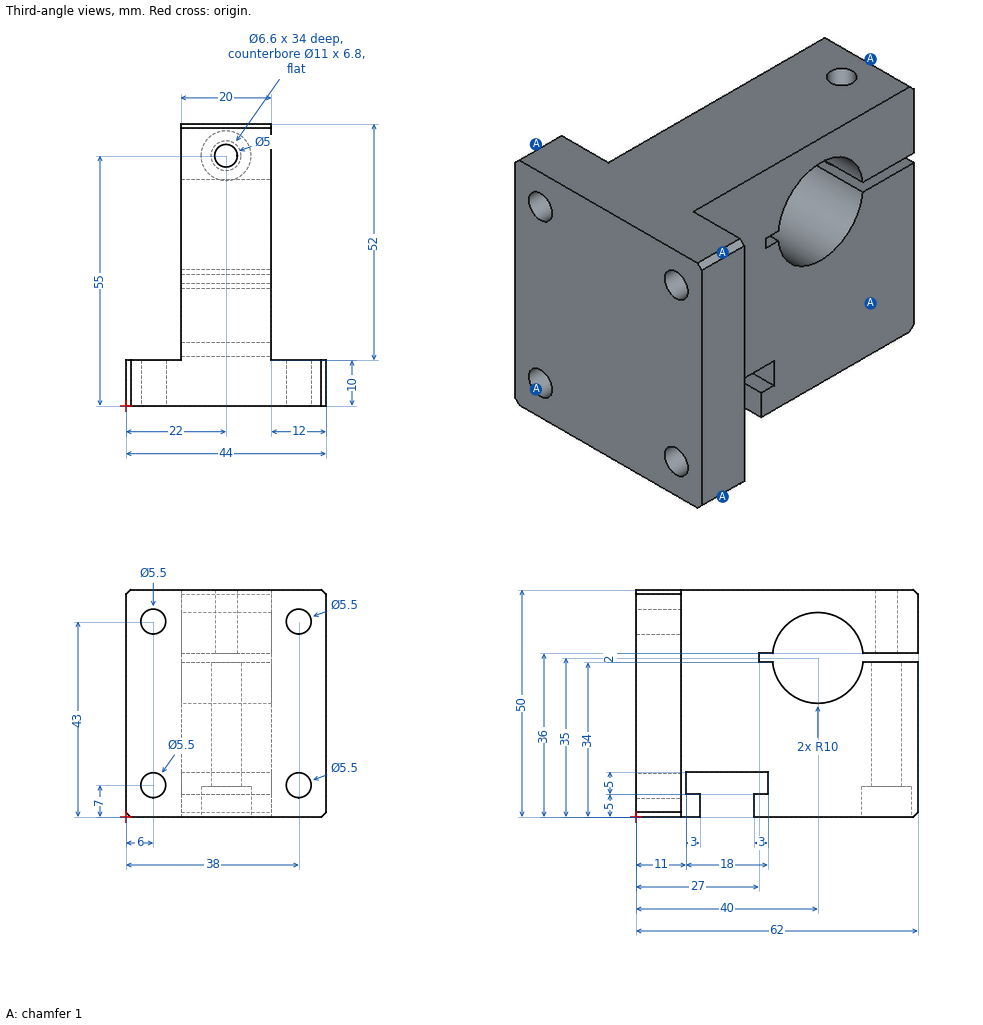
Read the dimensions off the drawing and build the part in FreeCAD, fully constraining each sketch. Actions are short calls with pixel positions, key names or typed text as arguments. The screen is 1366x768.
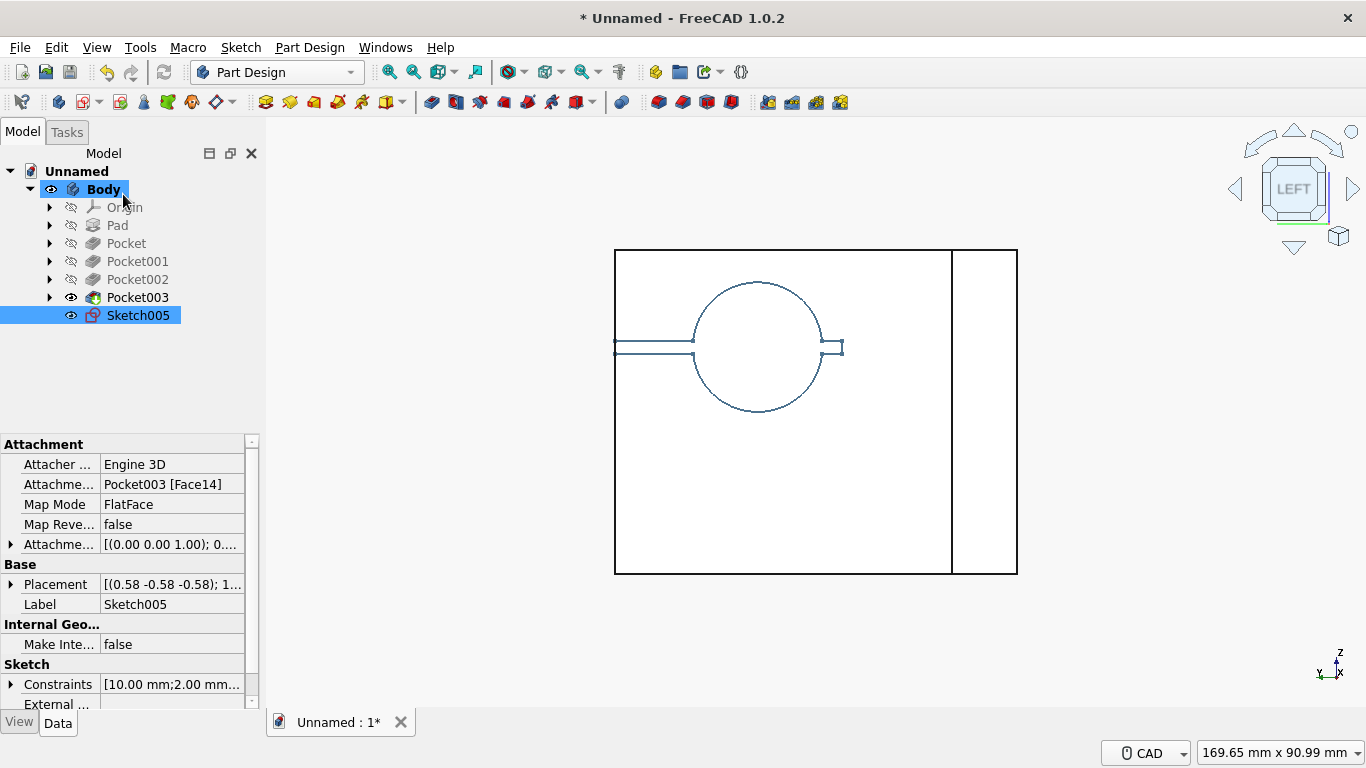
click(432, 102)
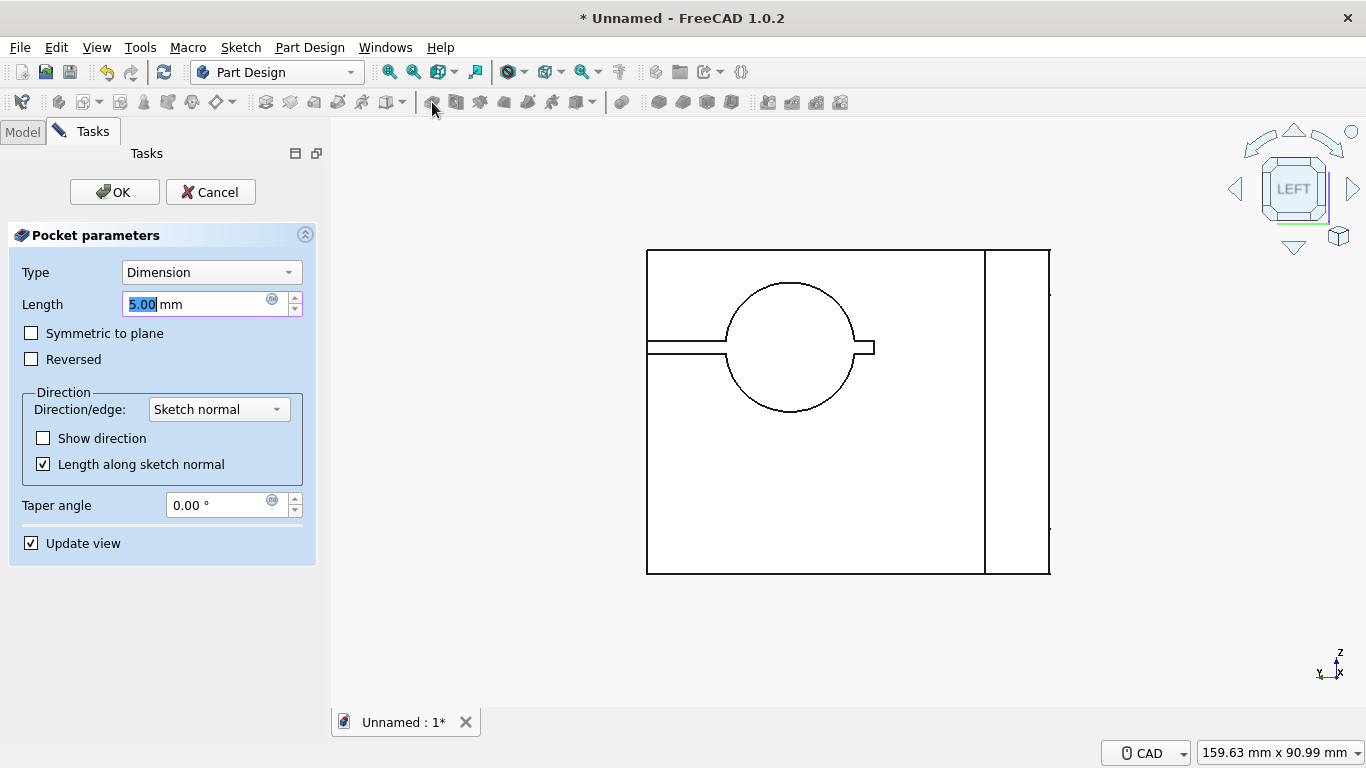
click(212, 272)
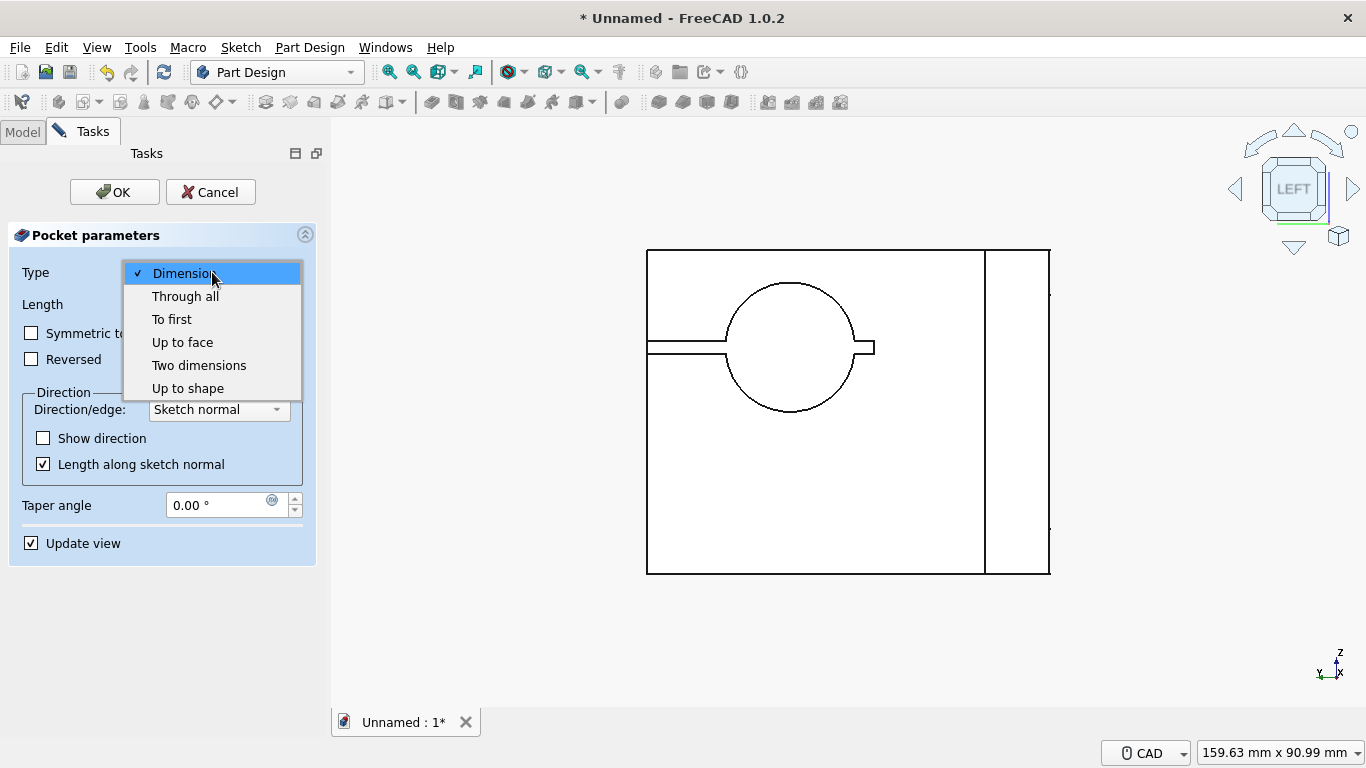
click(212, 320)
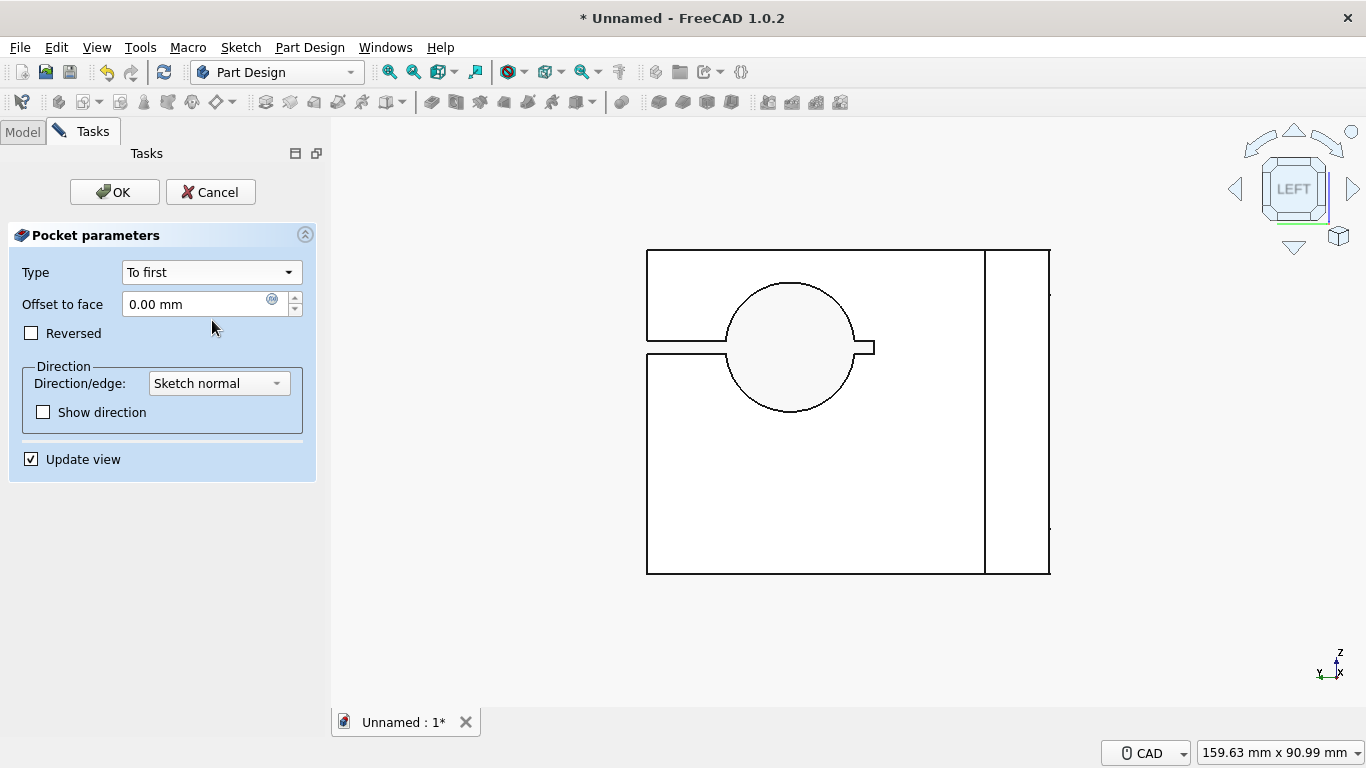
click(115, 192)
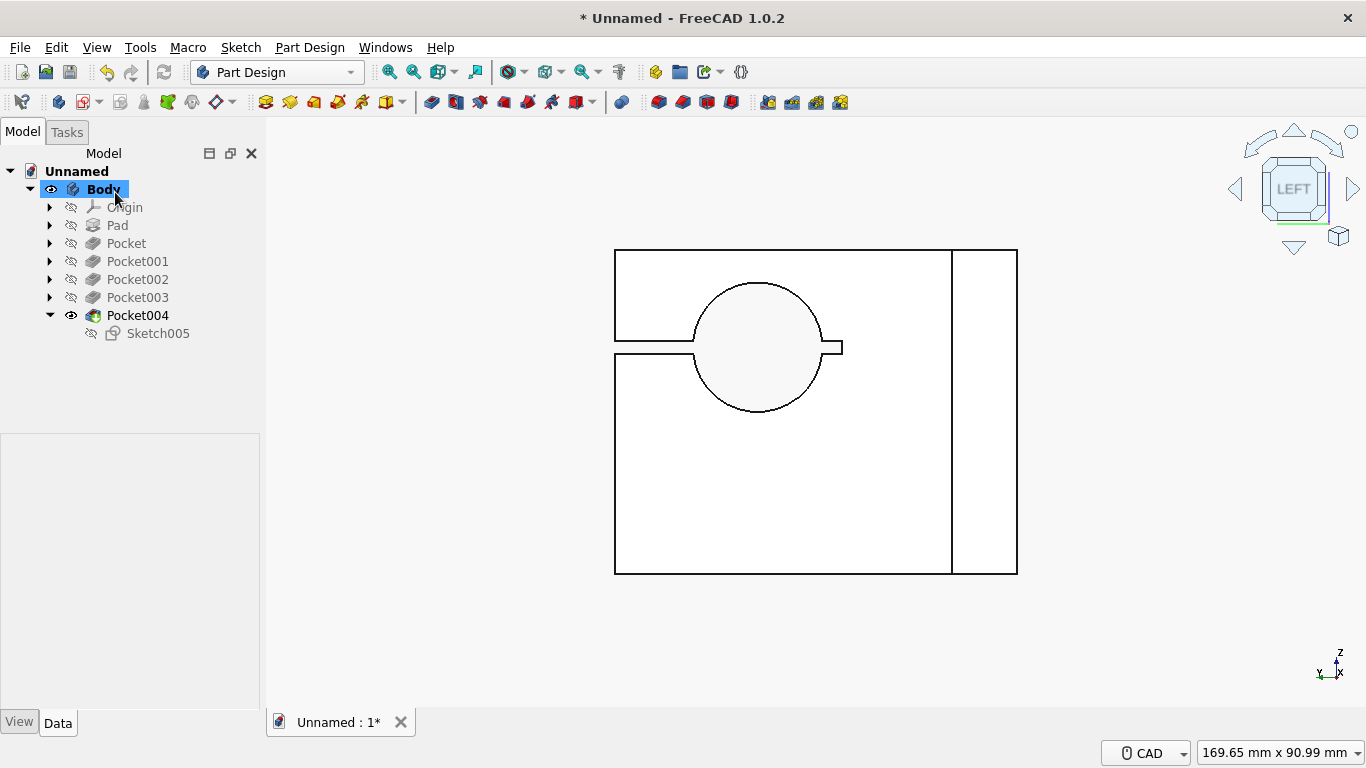
click(880, 457)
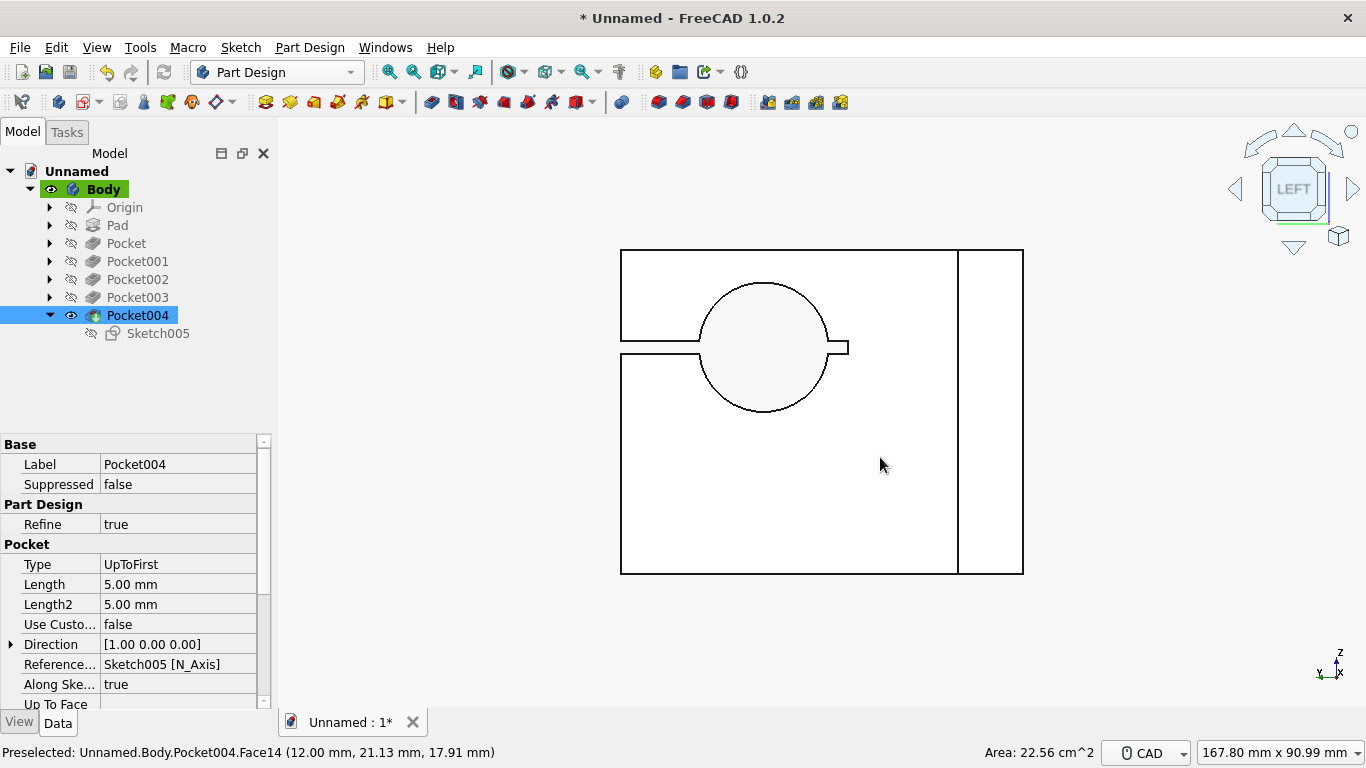
click(84, 102)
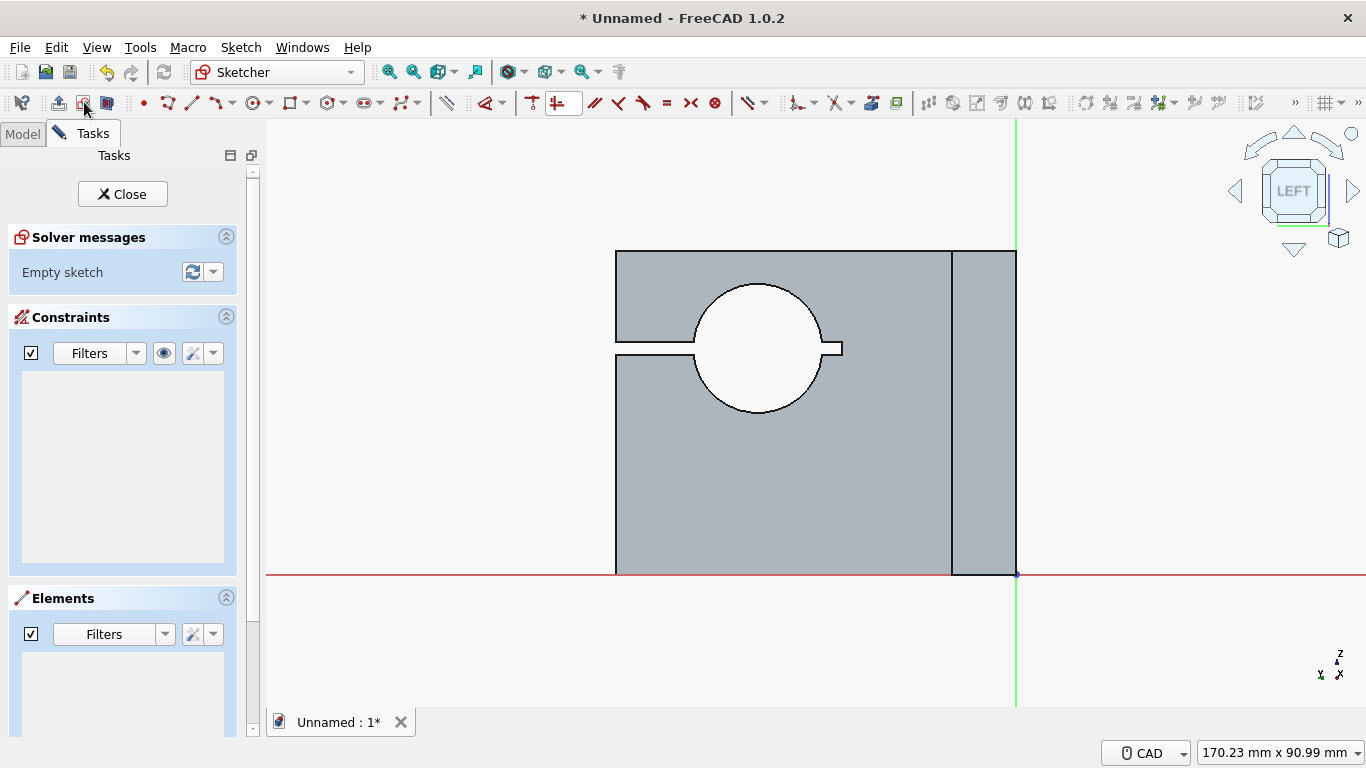
scroll(998, 598, up, 6)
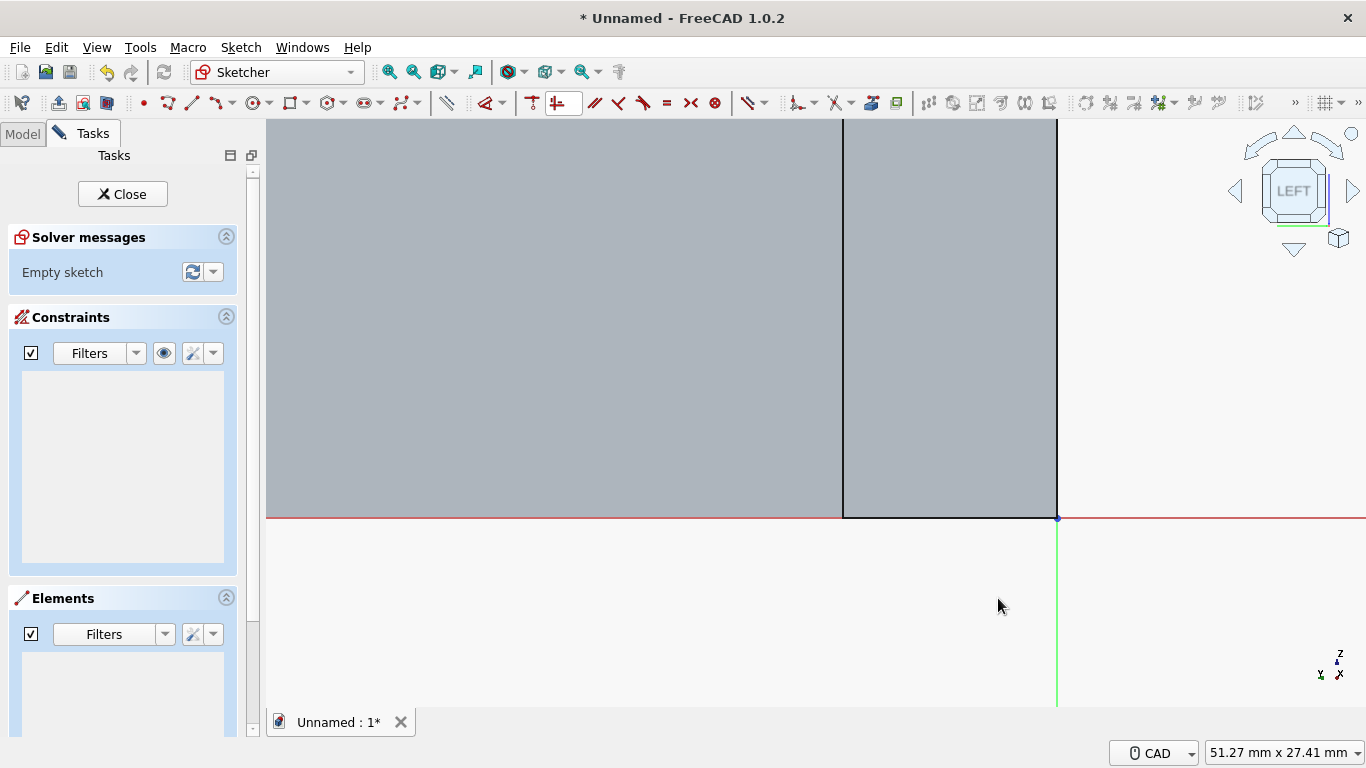
click(168, 104)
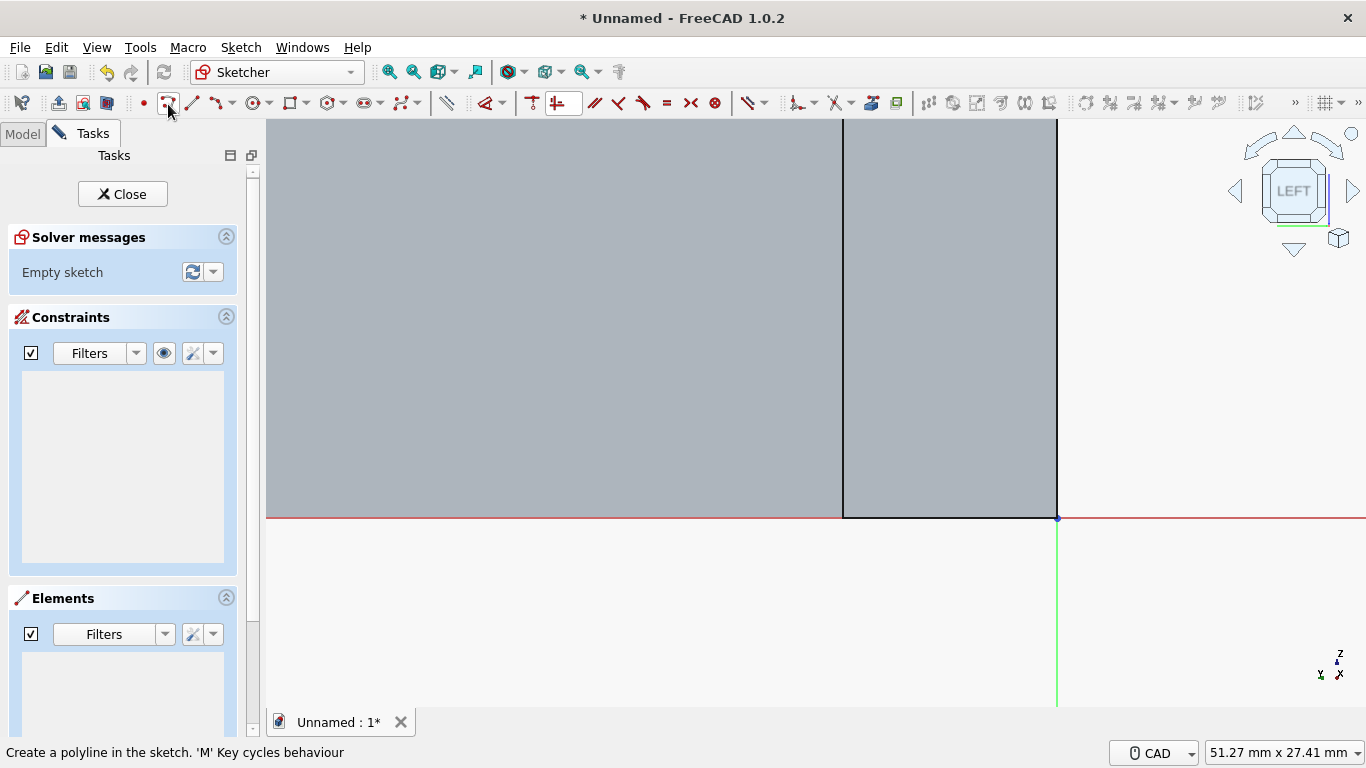
click(821, 411)
click(821, 304)
click(435, 304)
click(435, 411)
click(499, 411)
click(499, 518)
click(757, 509)
click(757, 411)
click(821, 412)
key(Escape)
key(Escape)